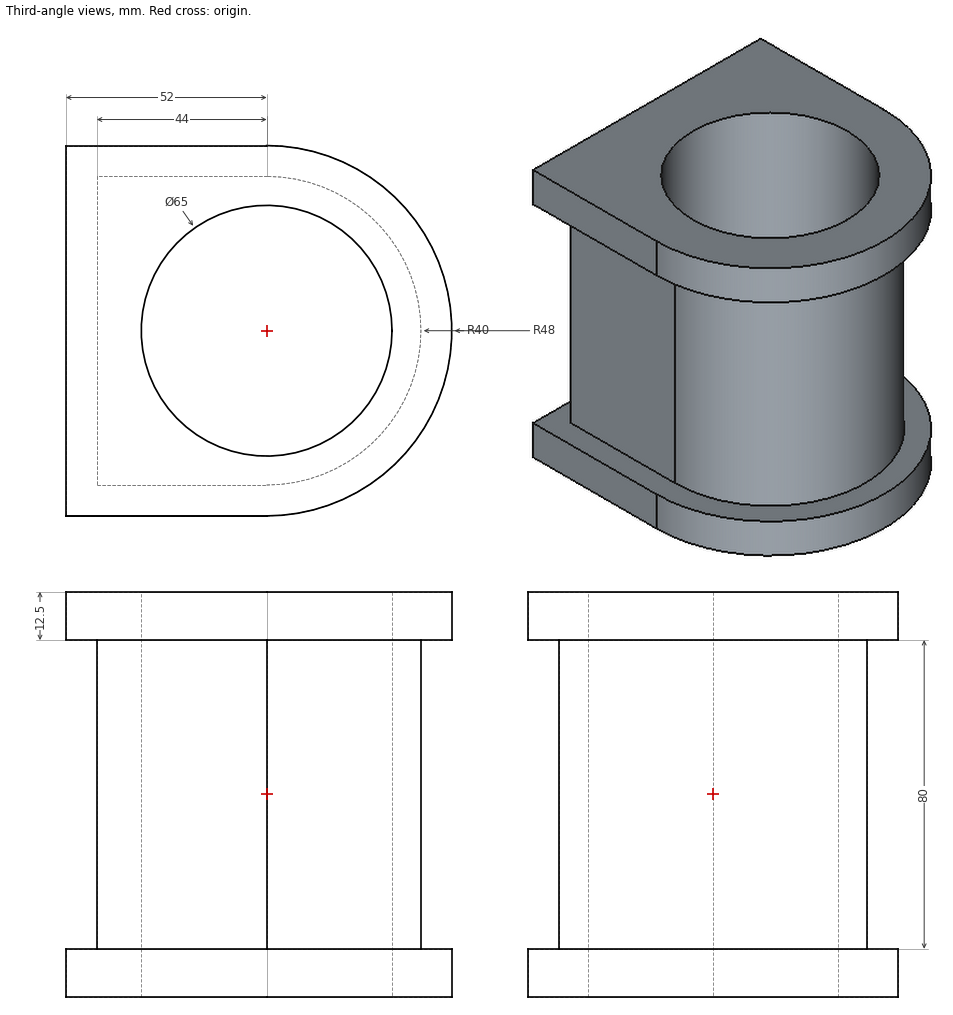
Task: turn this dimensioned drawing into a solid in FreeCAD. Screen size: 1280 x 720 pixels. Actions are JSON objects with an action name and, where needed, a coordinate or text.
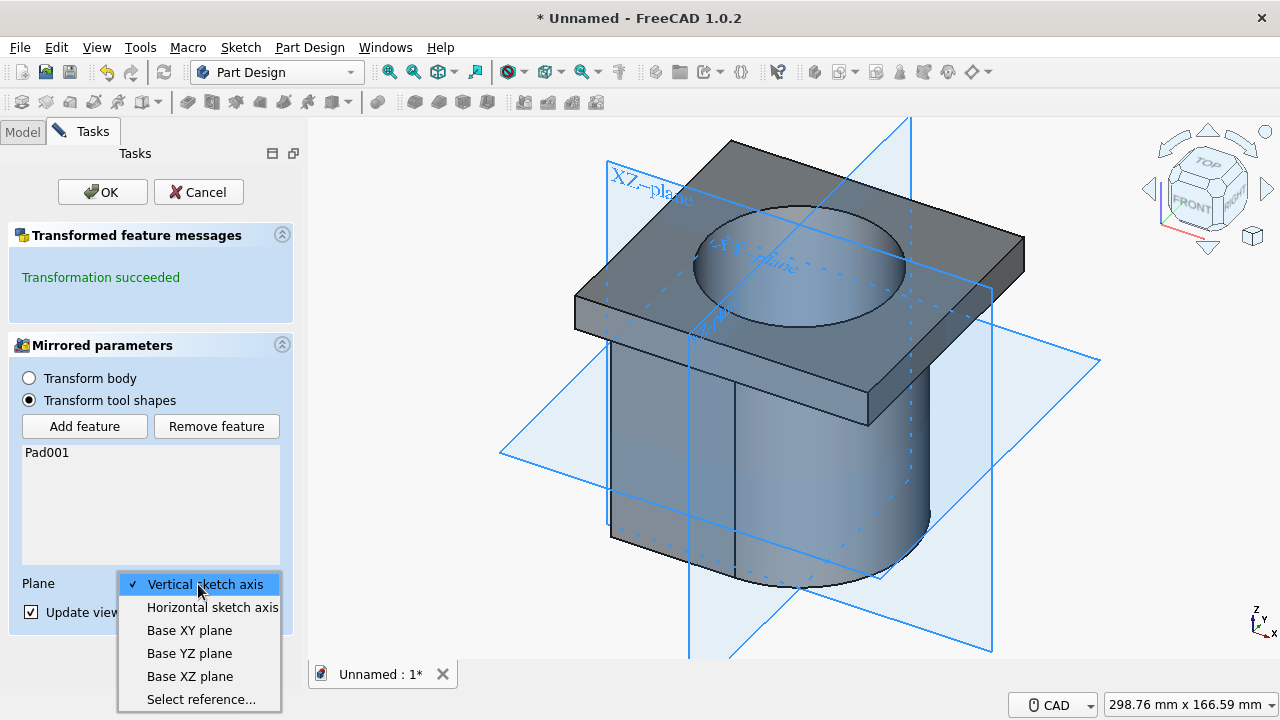
{"action": "left_click", "coordinate": [198, 630]}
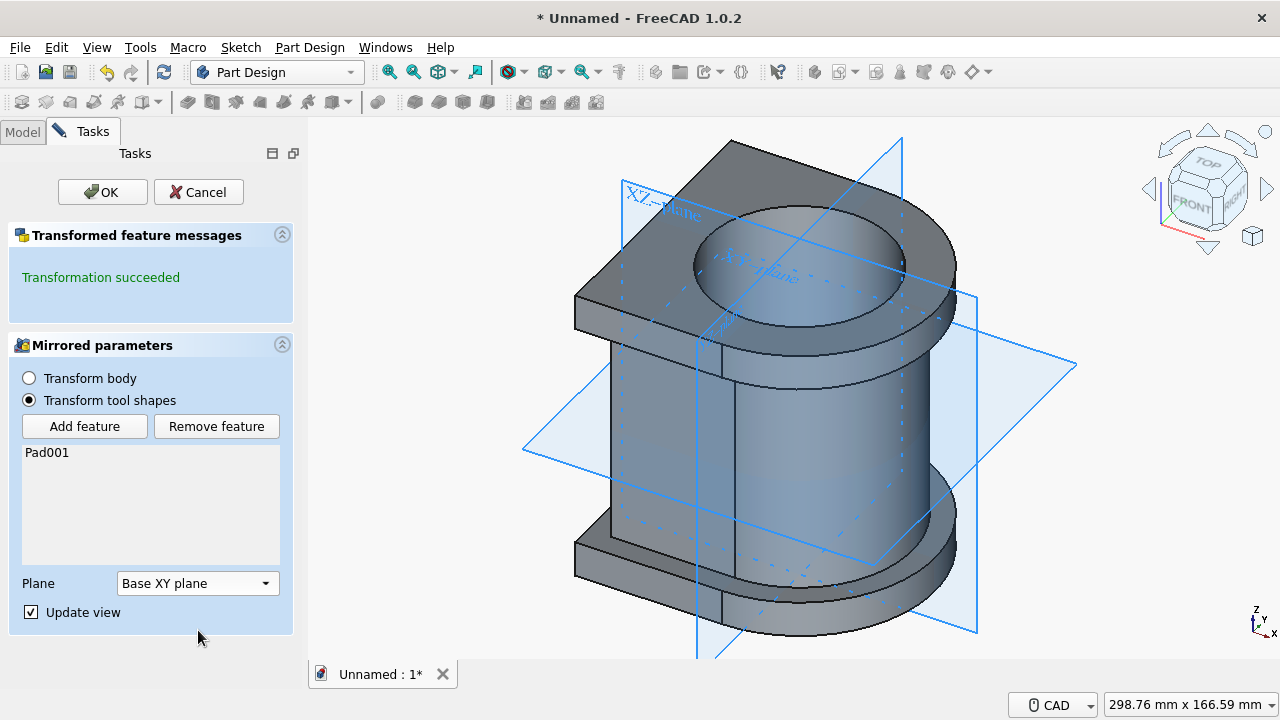
{"action": "left_click", "coordinate": [103, 192]}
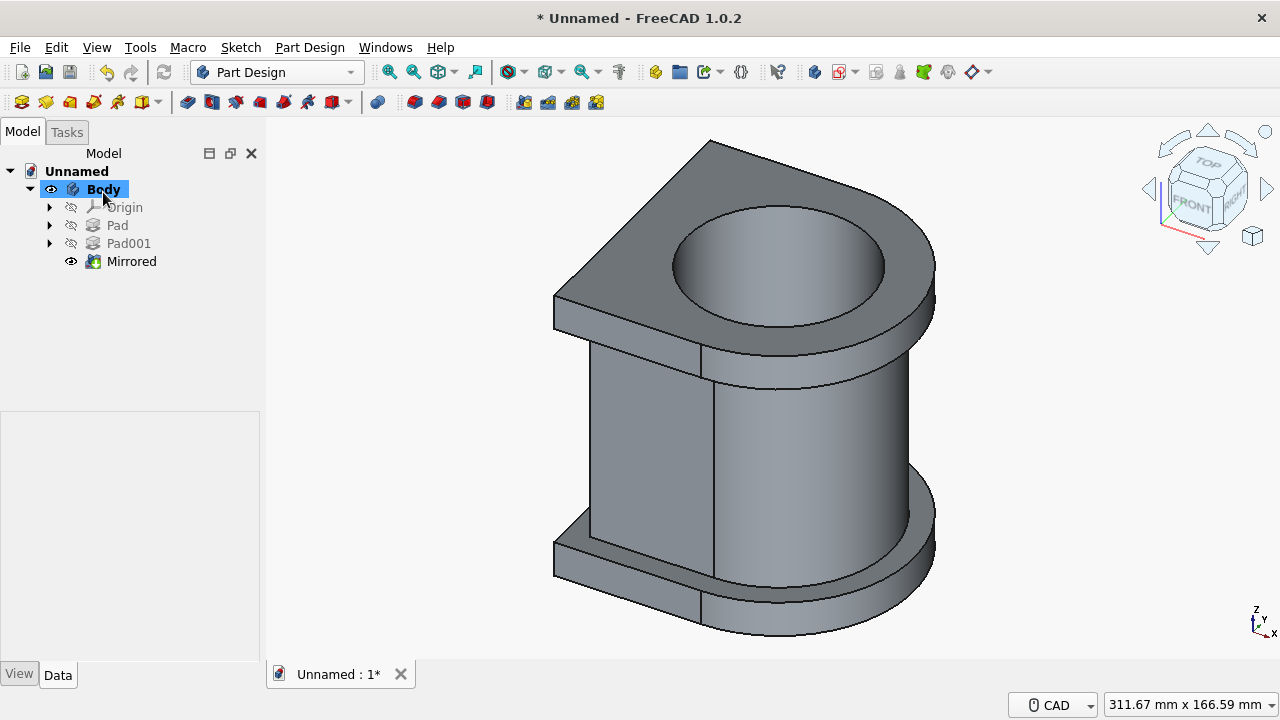
{"action": "key", "text": "0"}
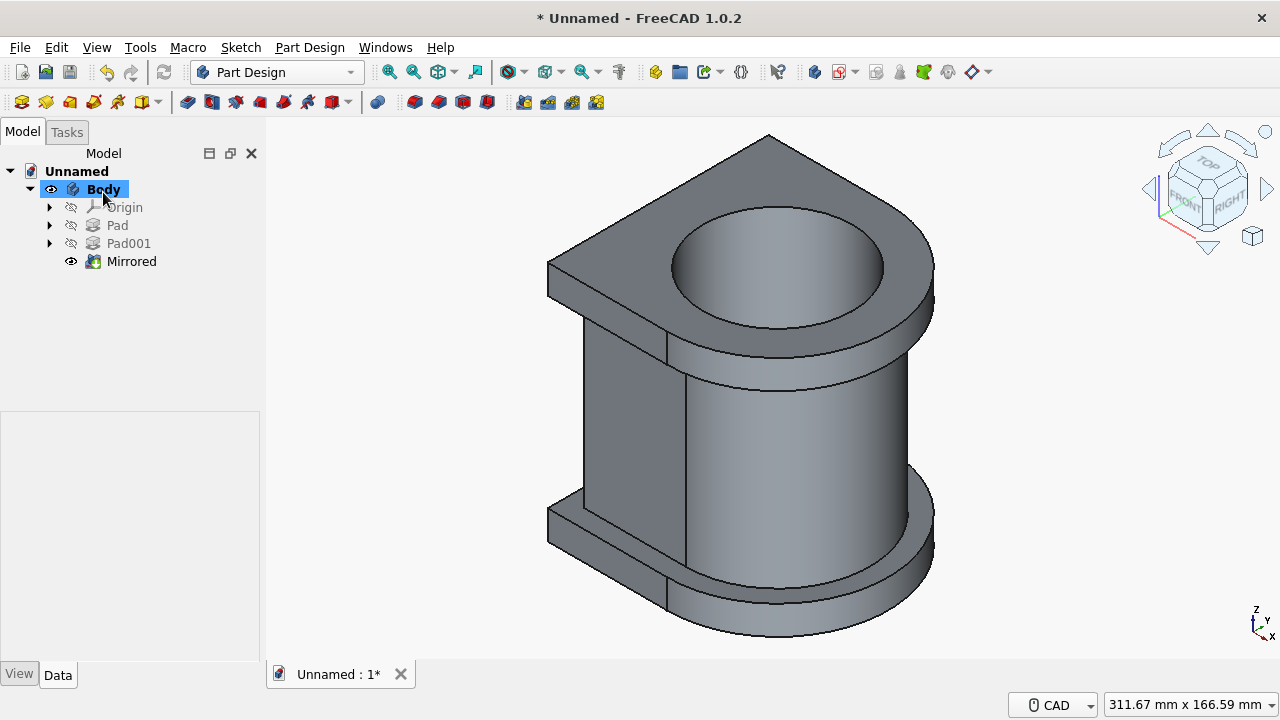
{"action": "left_click", "coordinate": [390, 72]}